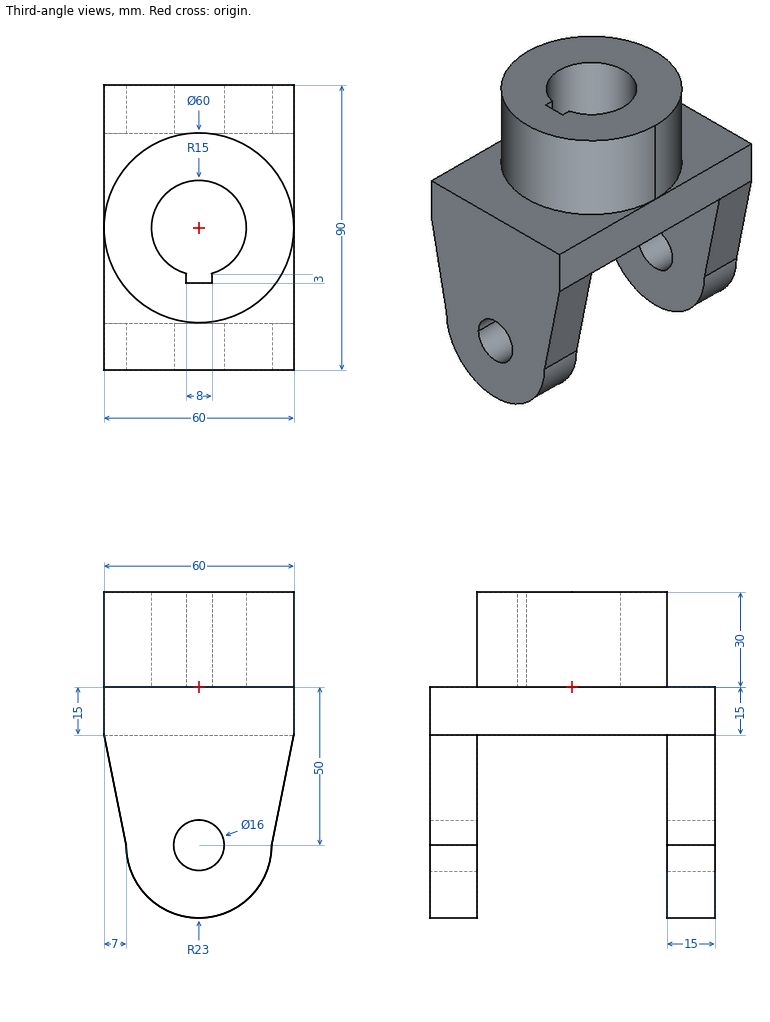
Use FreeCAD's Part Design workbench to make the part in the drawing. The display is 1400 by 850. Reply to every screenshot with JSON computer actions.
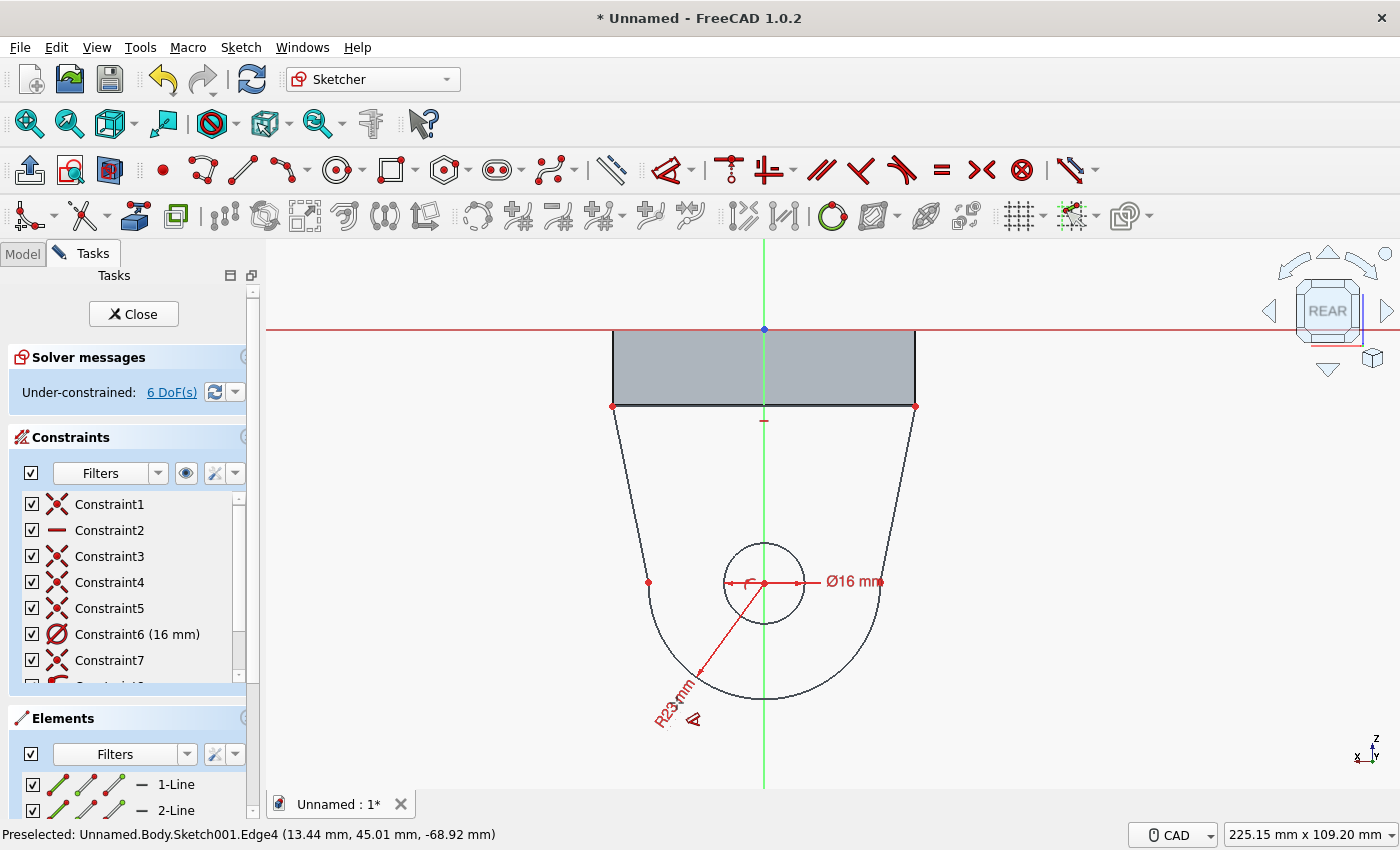
{"action": "left_click", "coordinate": [825, 406]}
{"action": "left_click", "coordinate": [695, 372]}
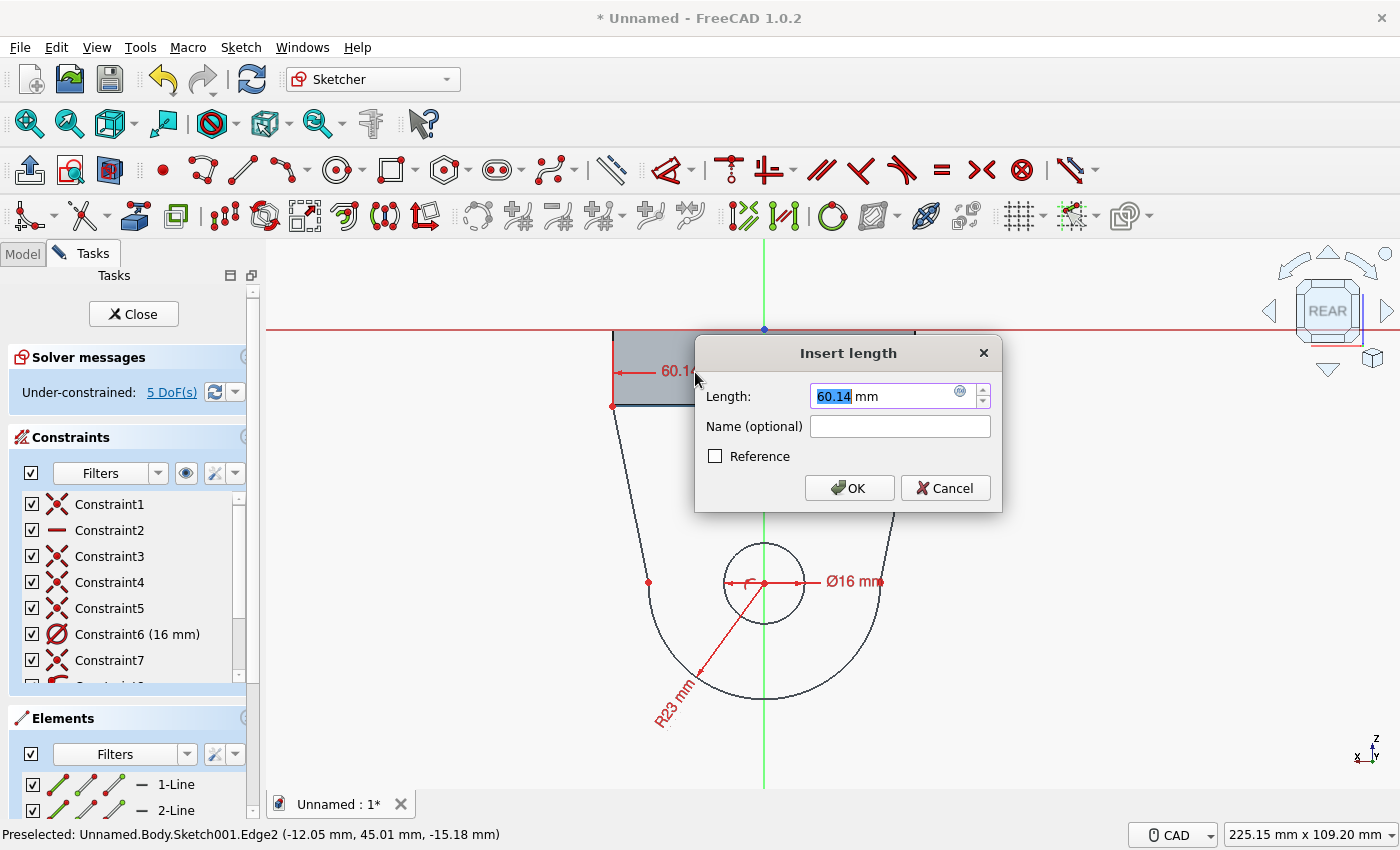
{"action": "type", "text": "60"}
{"action": "key", "text": "Return"}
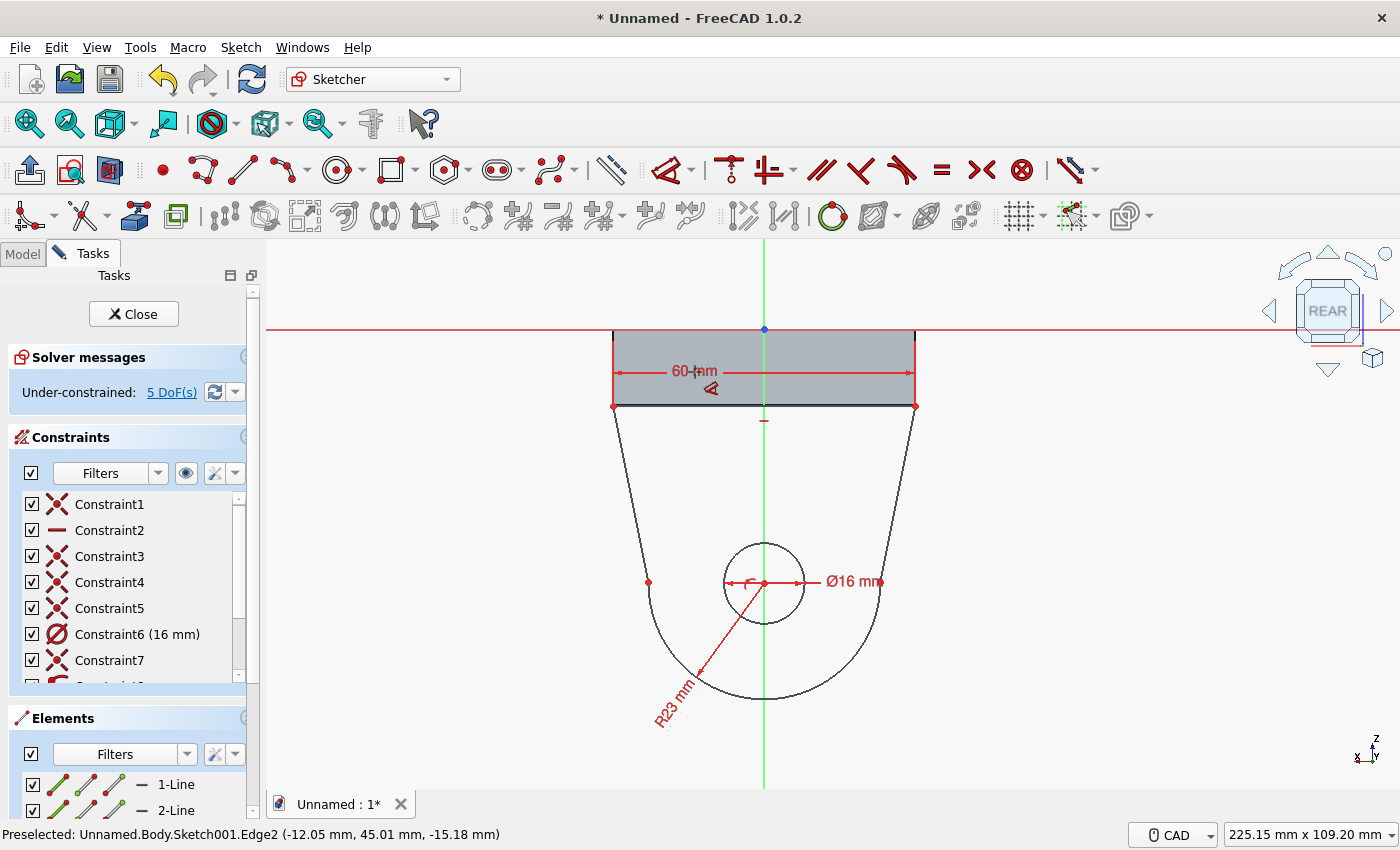
{"action": "left_click", "coordinate": [891, 530]}
{"action": "left_click", "coordinate": [898, 372]}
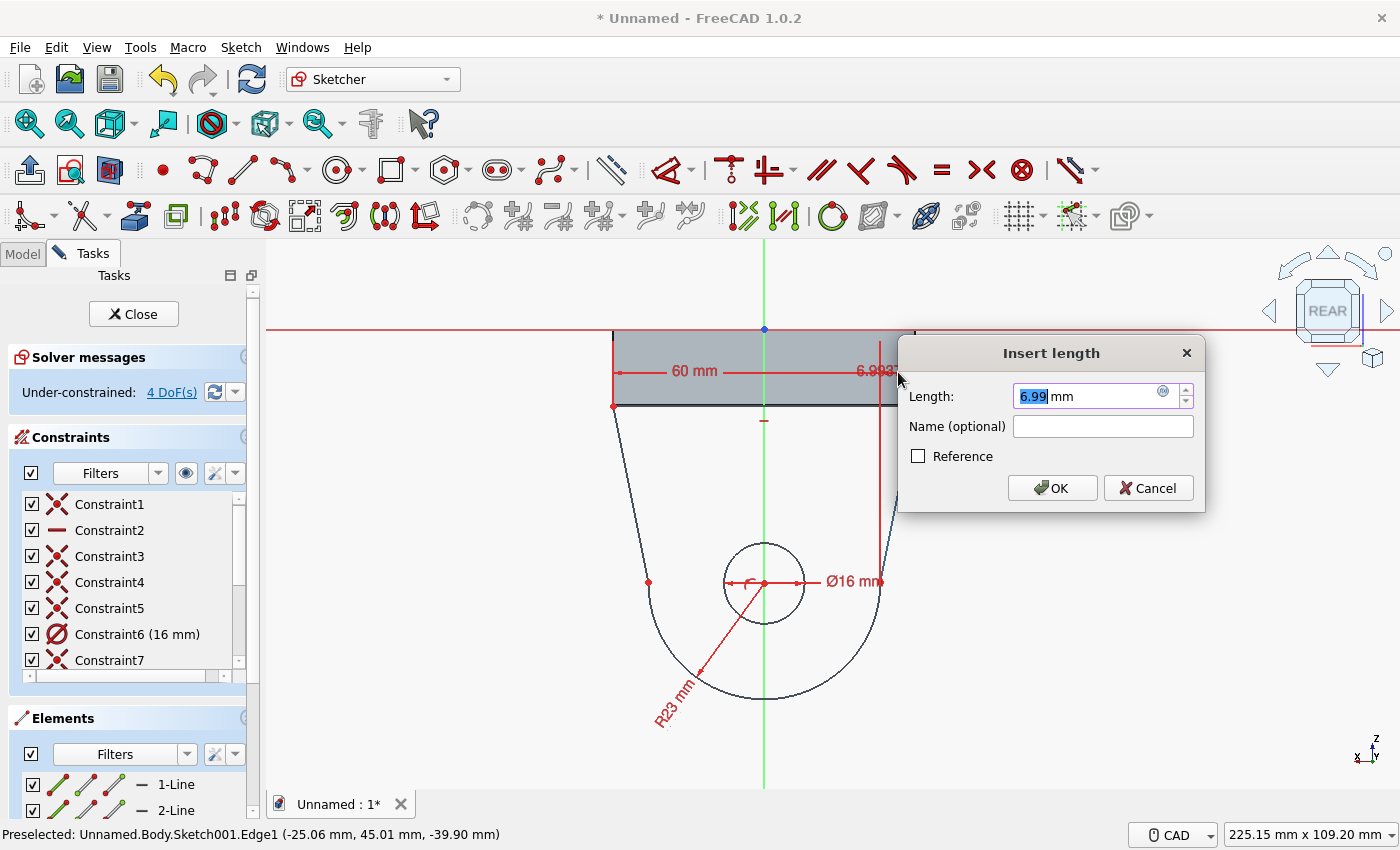
{"action": "type", "text": "7"}
{"action": "key", "text": "Return"}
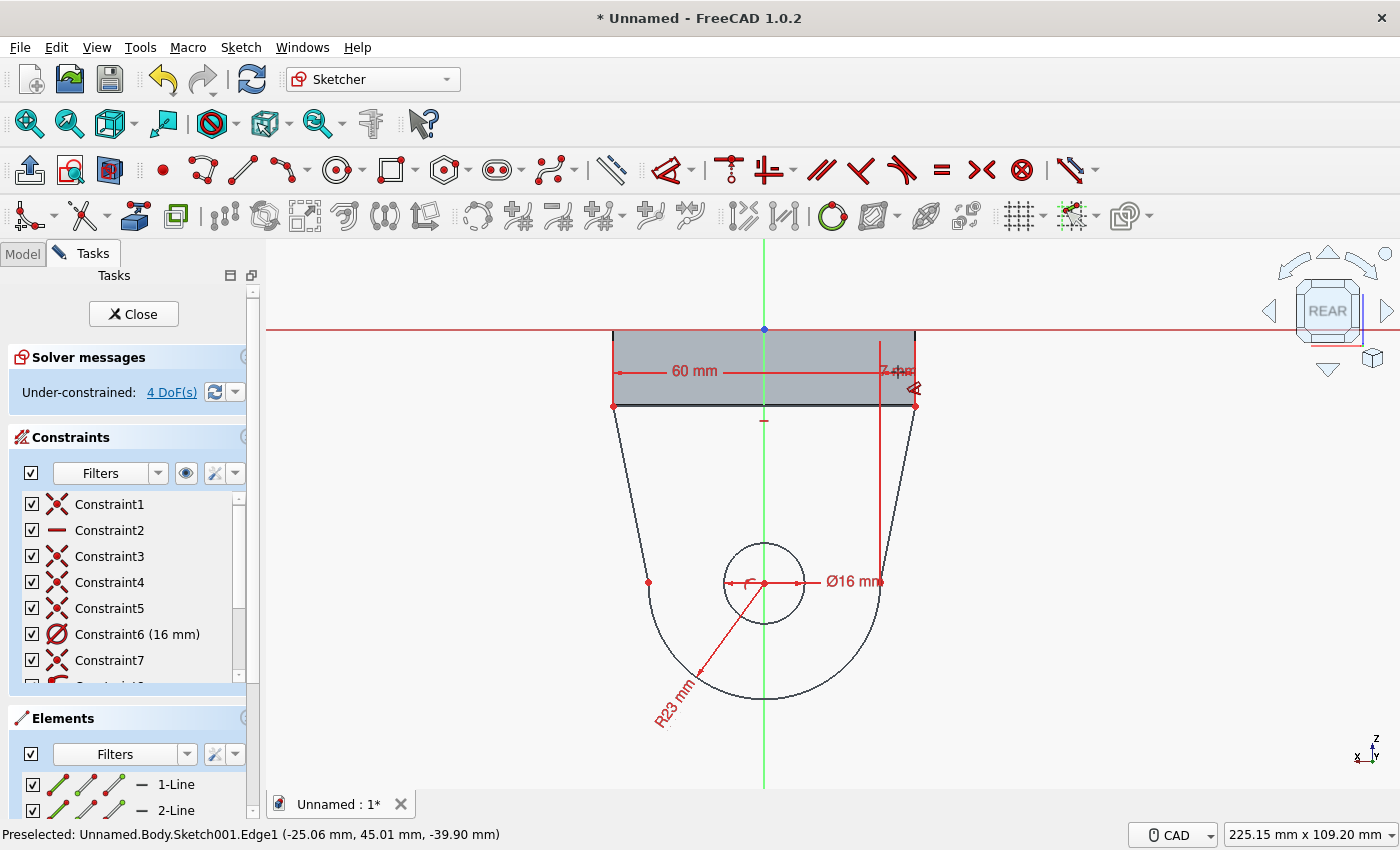
{"action": "left_click", "coordinate": [764, 583]}
{"action": "left_click", "coordinate": [798, 457]}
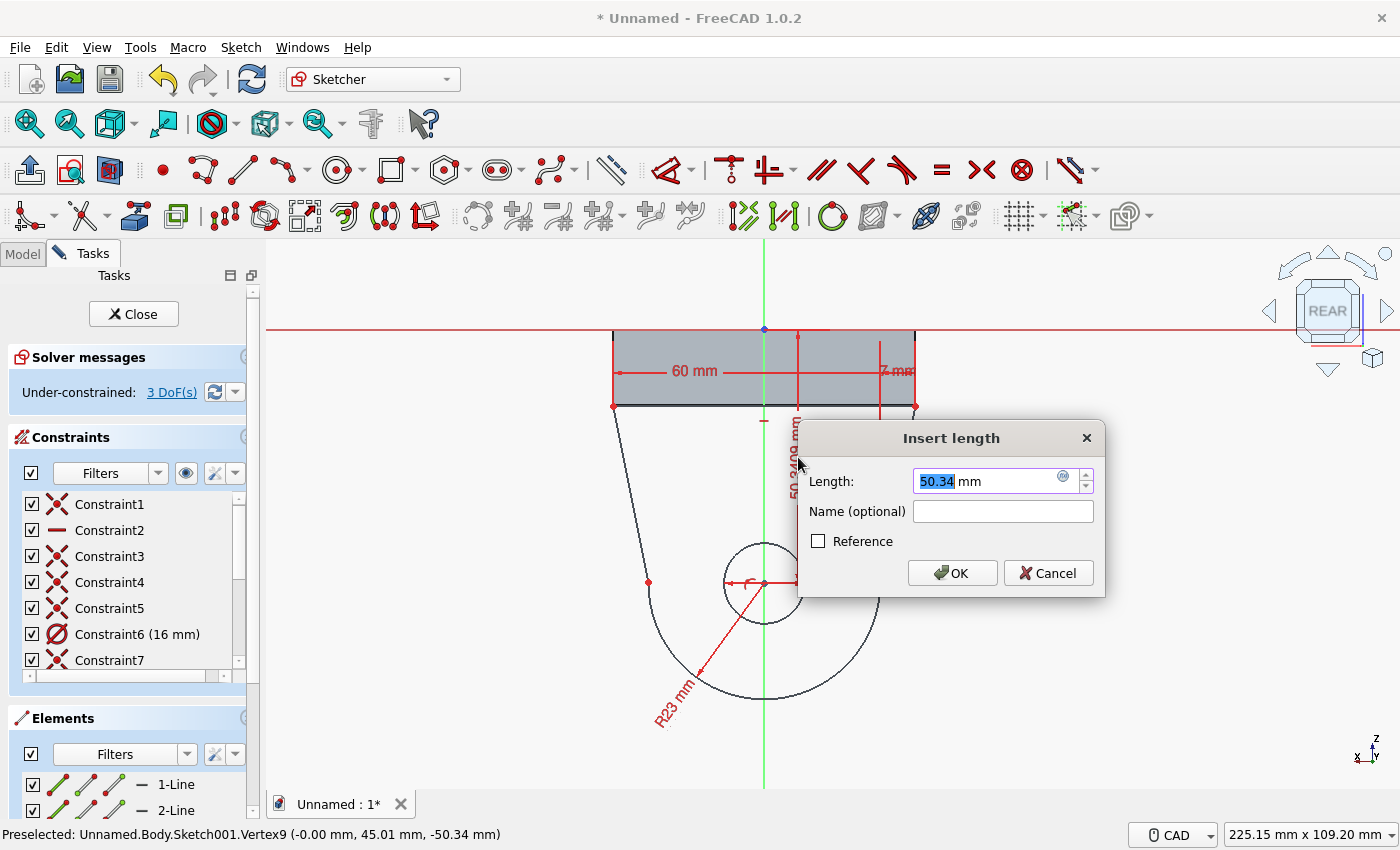
{"action": "type", "text": "50"}
{"action": "key", "text": "Return"}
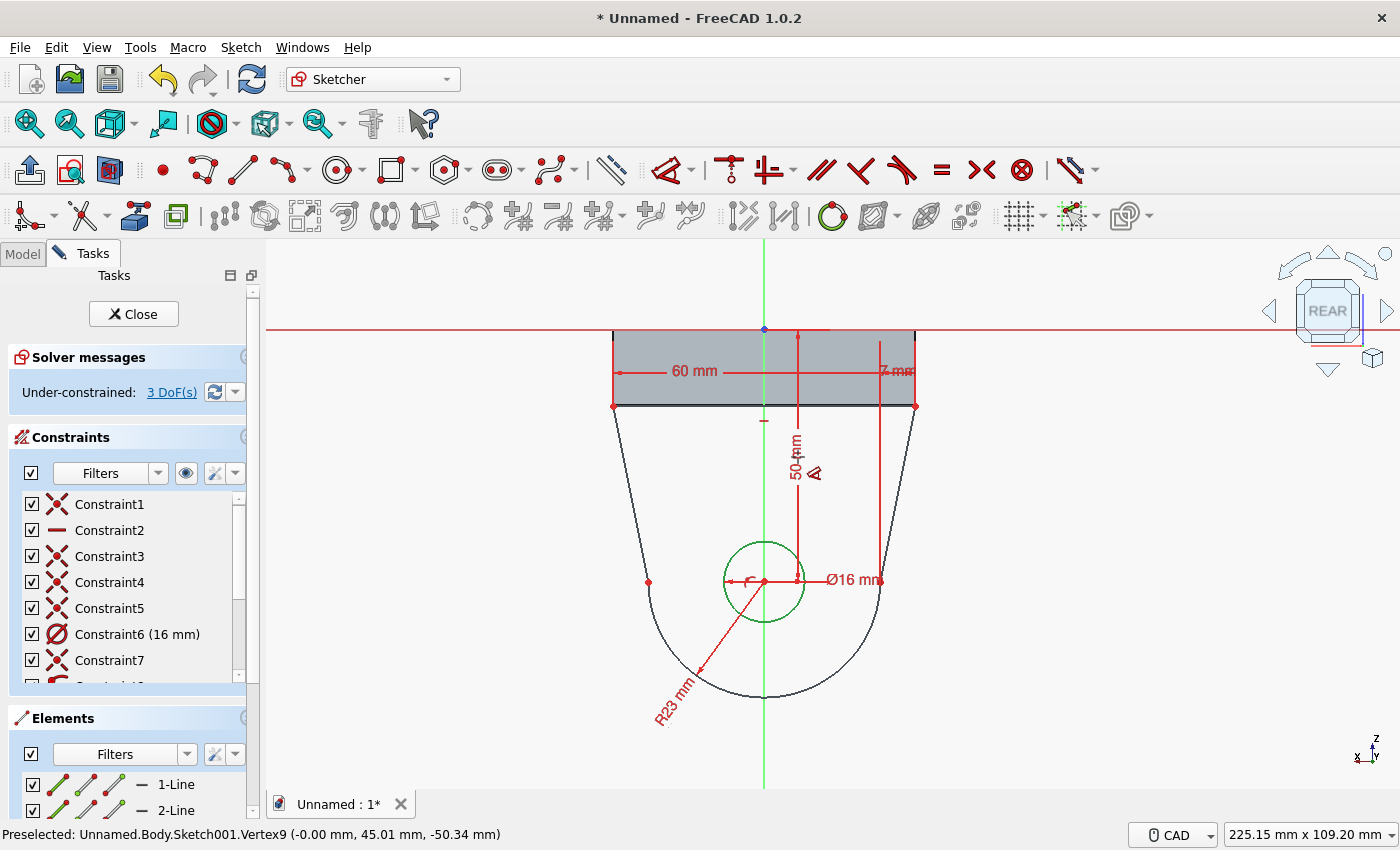
{"action": "left_click", "coordinate": [880, 583]}
{"action": "left_click", "coordinate": [914, 514]}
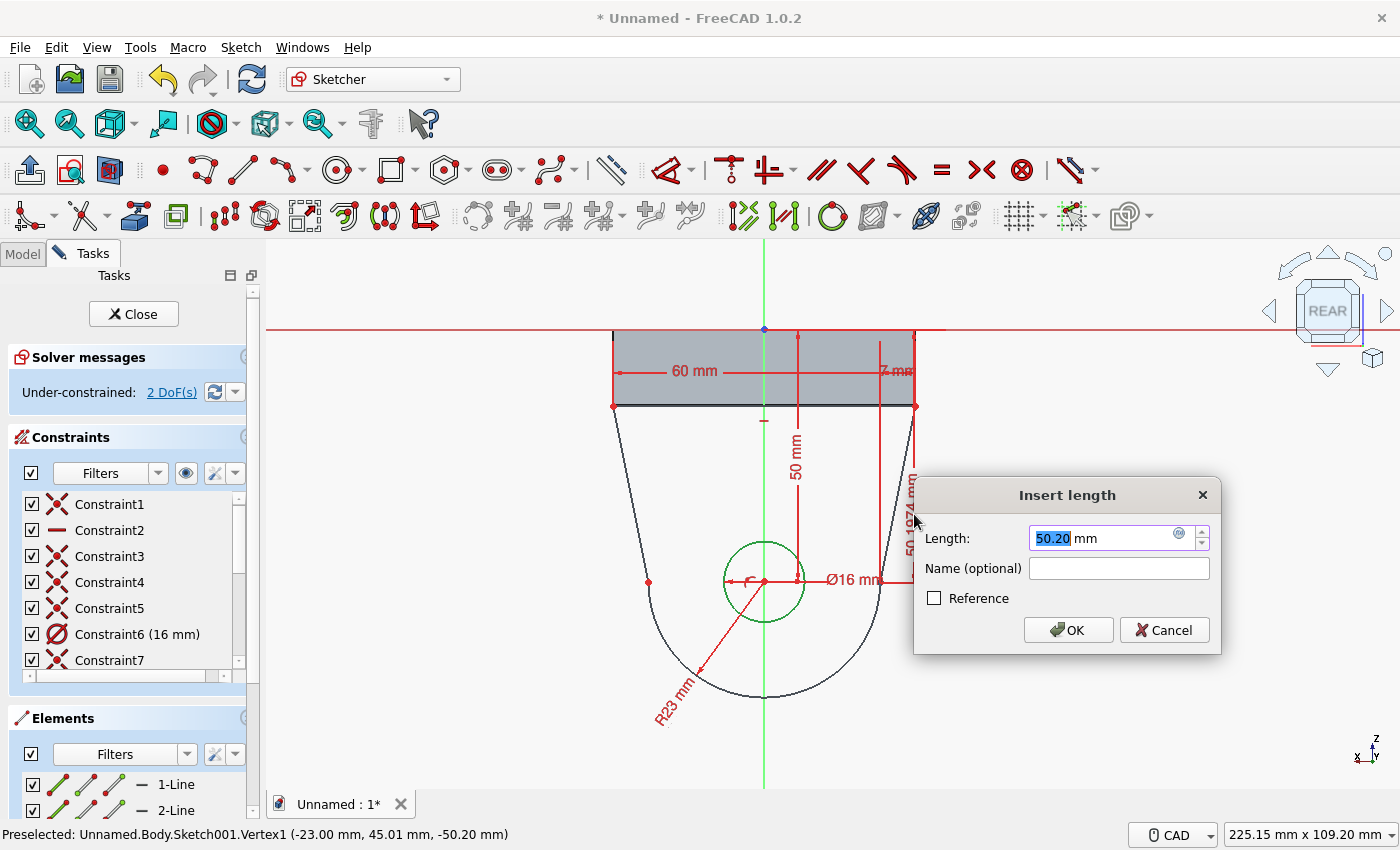
{"action": "type", "text": "50"}
{"action": "key", "text": "Return"}